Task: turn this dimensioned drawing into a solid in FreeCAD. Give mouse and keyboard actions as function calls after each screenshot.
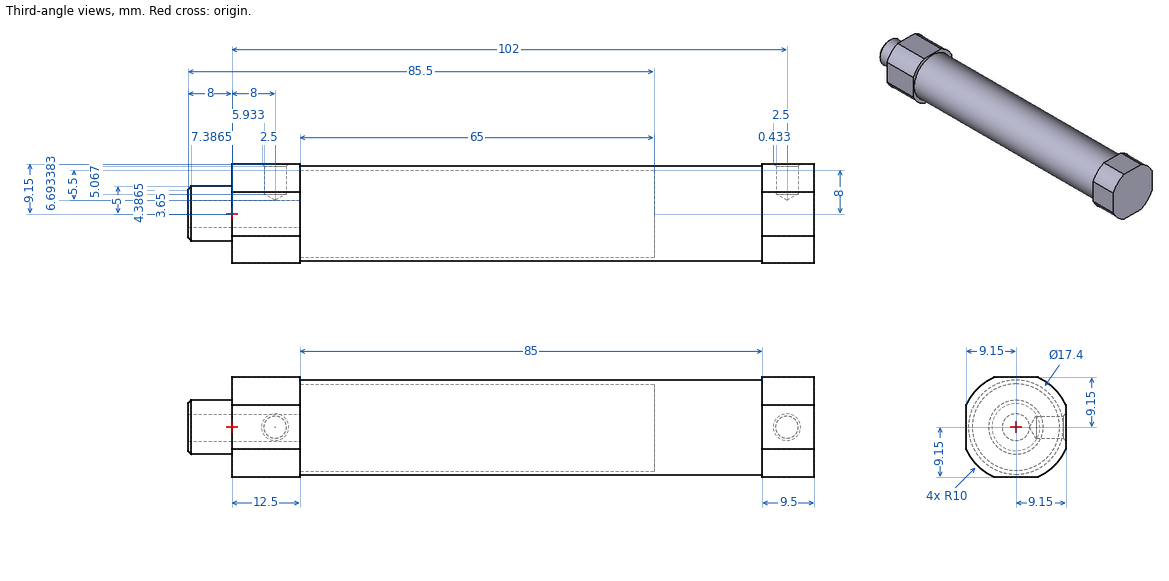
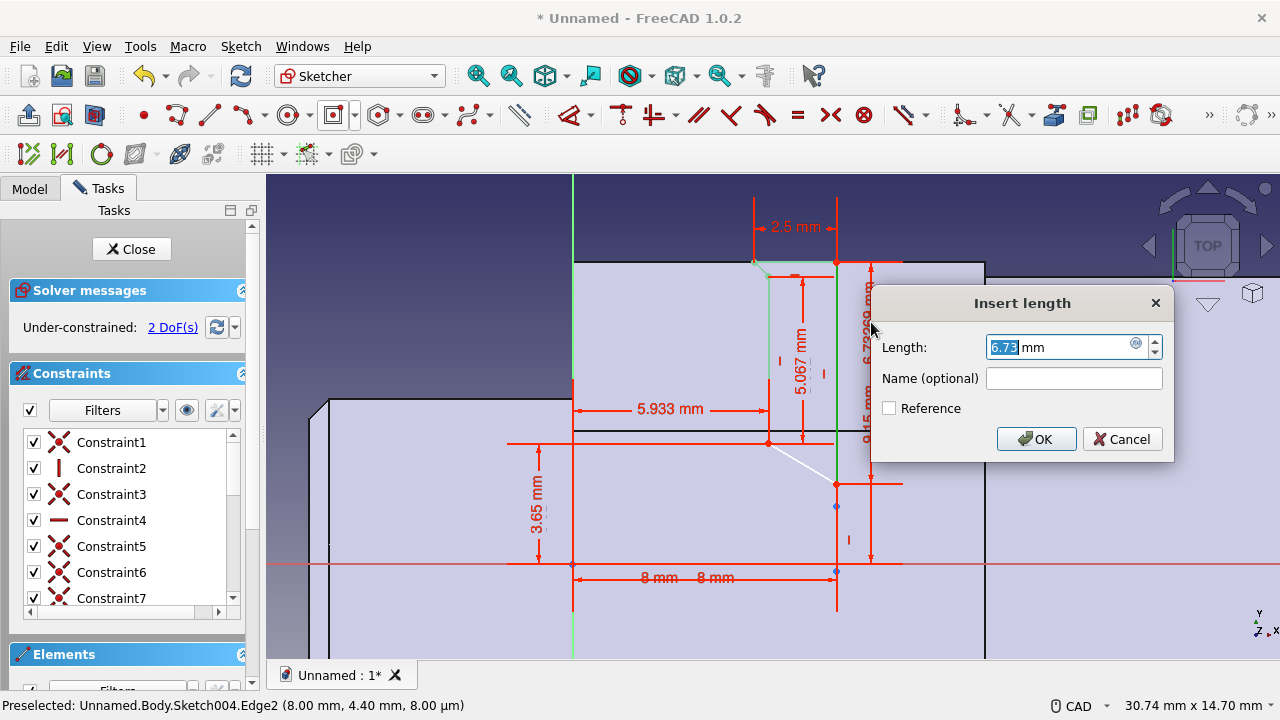
text(6.693383)
key(Return)
key(Escape)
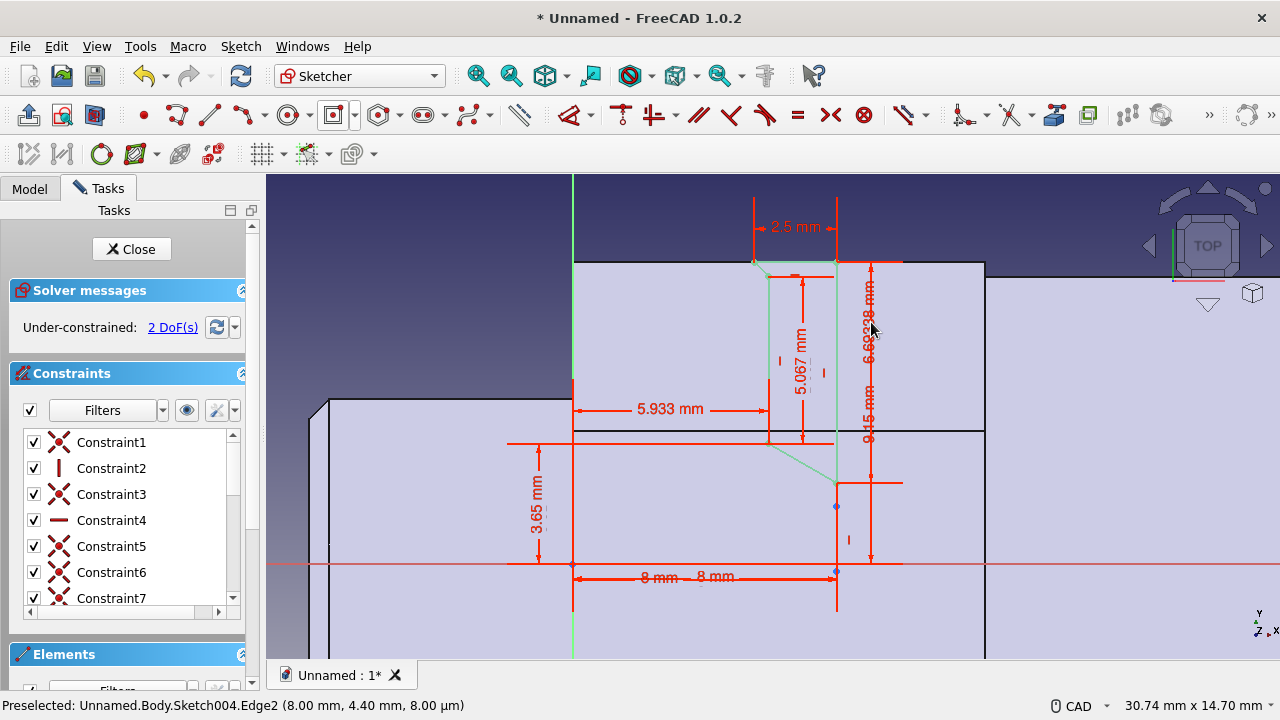
click(132, 249)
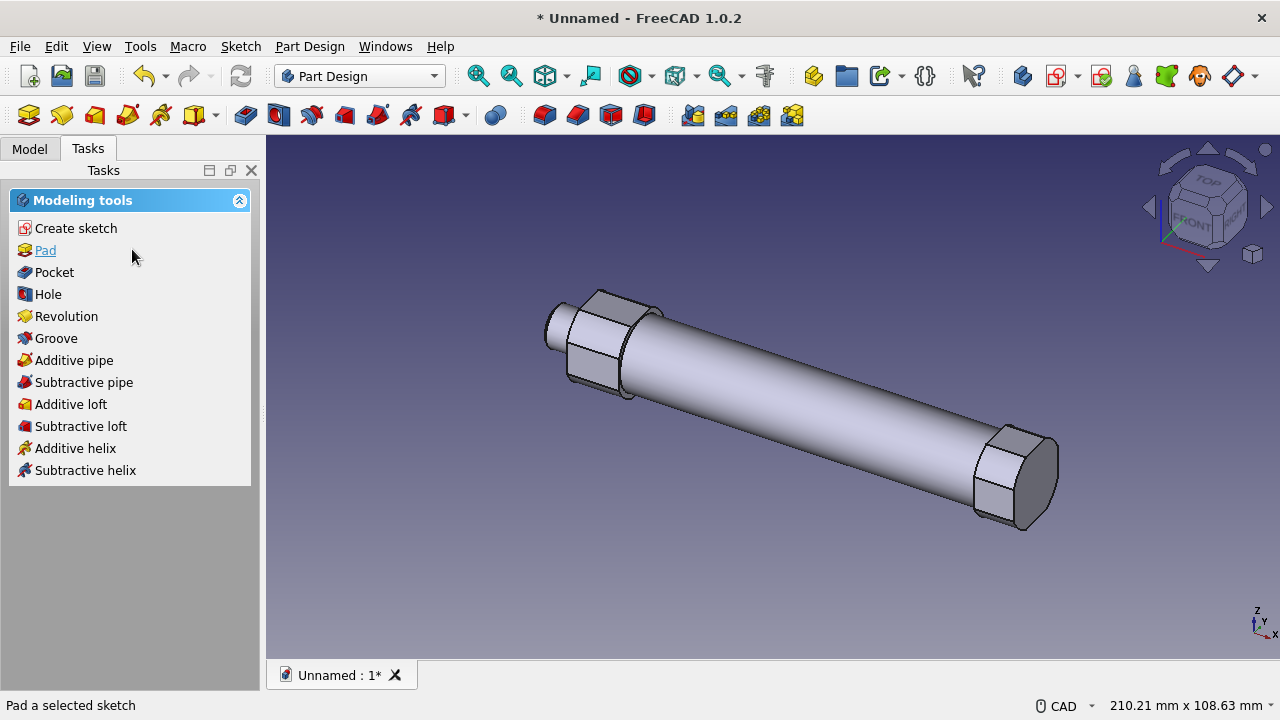
click(312, 116)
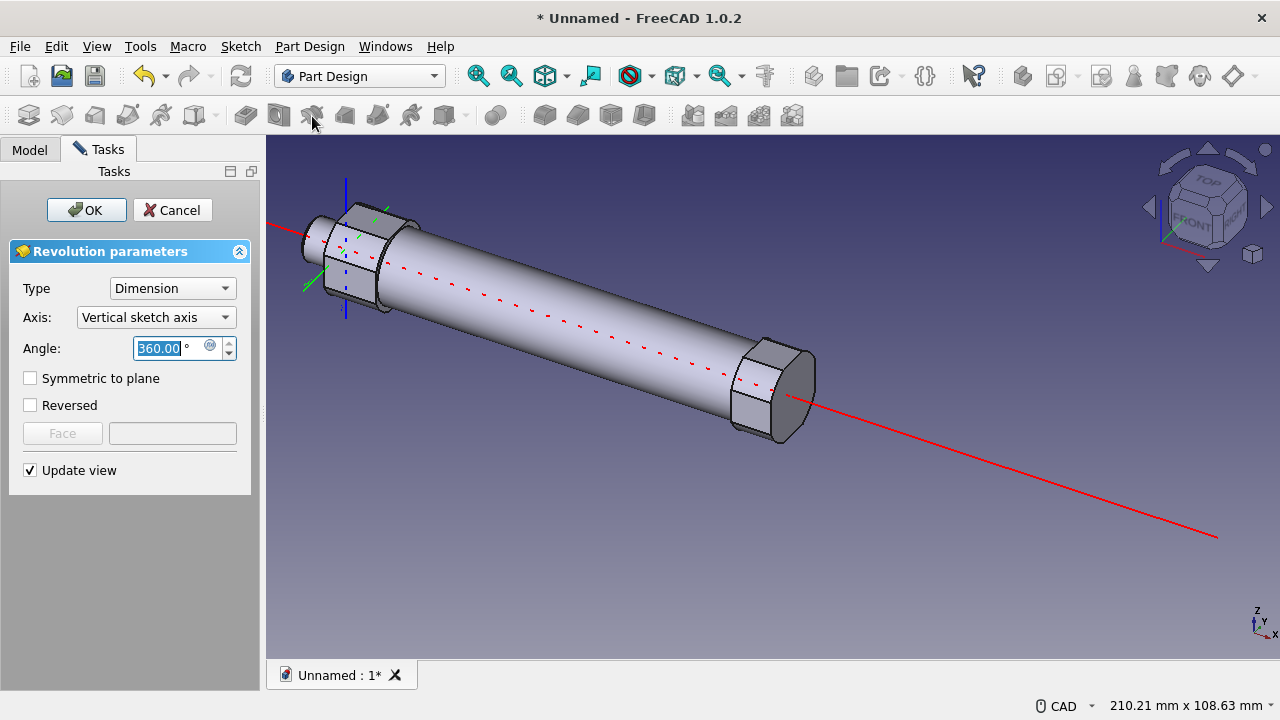
click(157, 318)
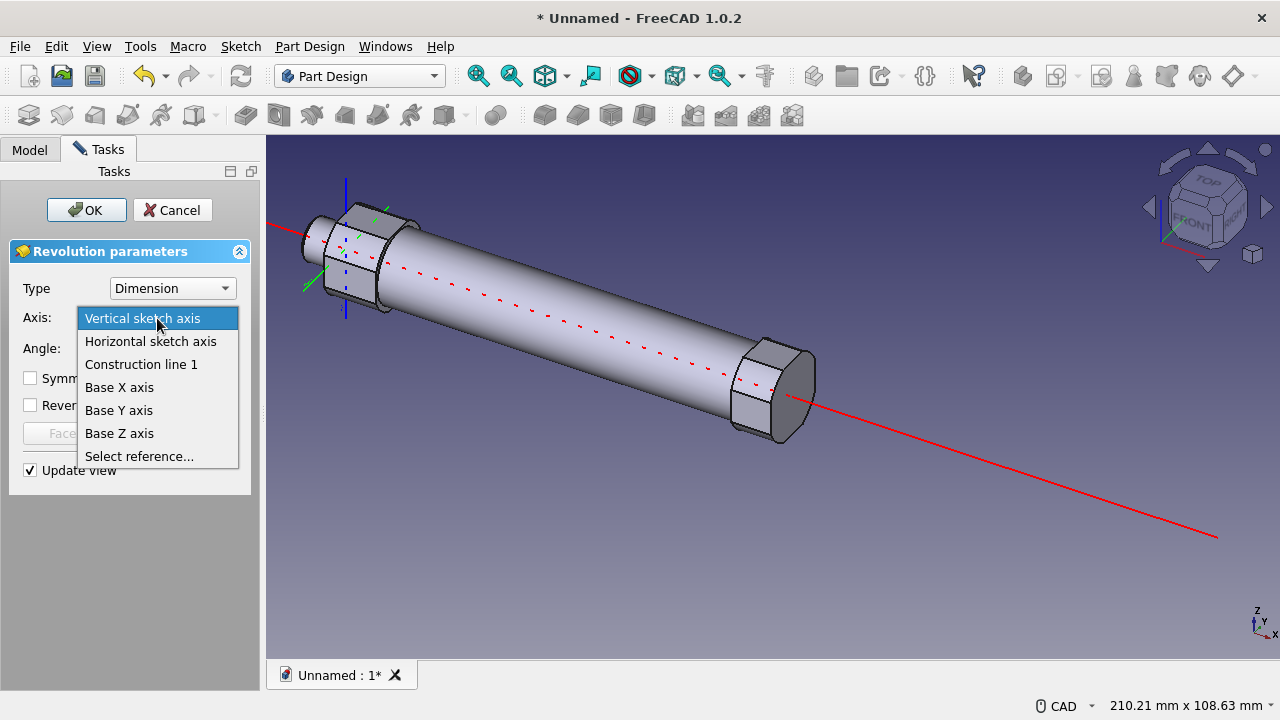
click(156, 364)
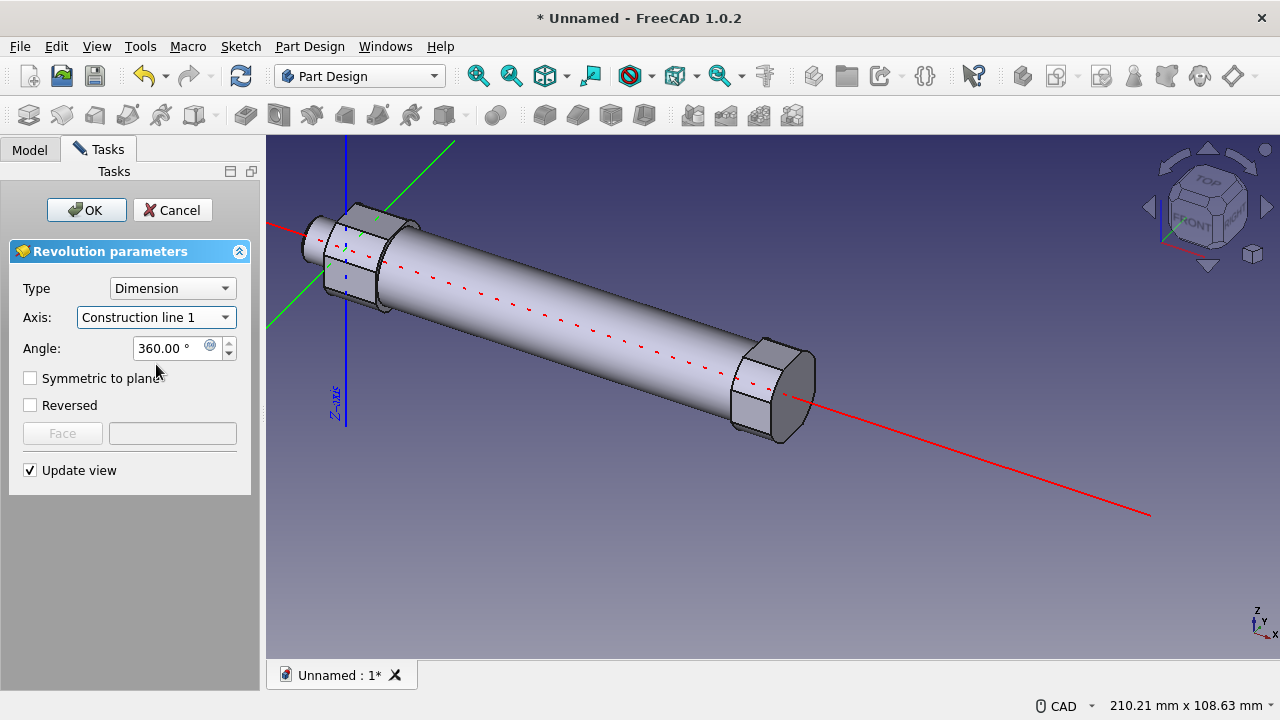
click(87, 210)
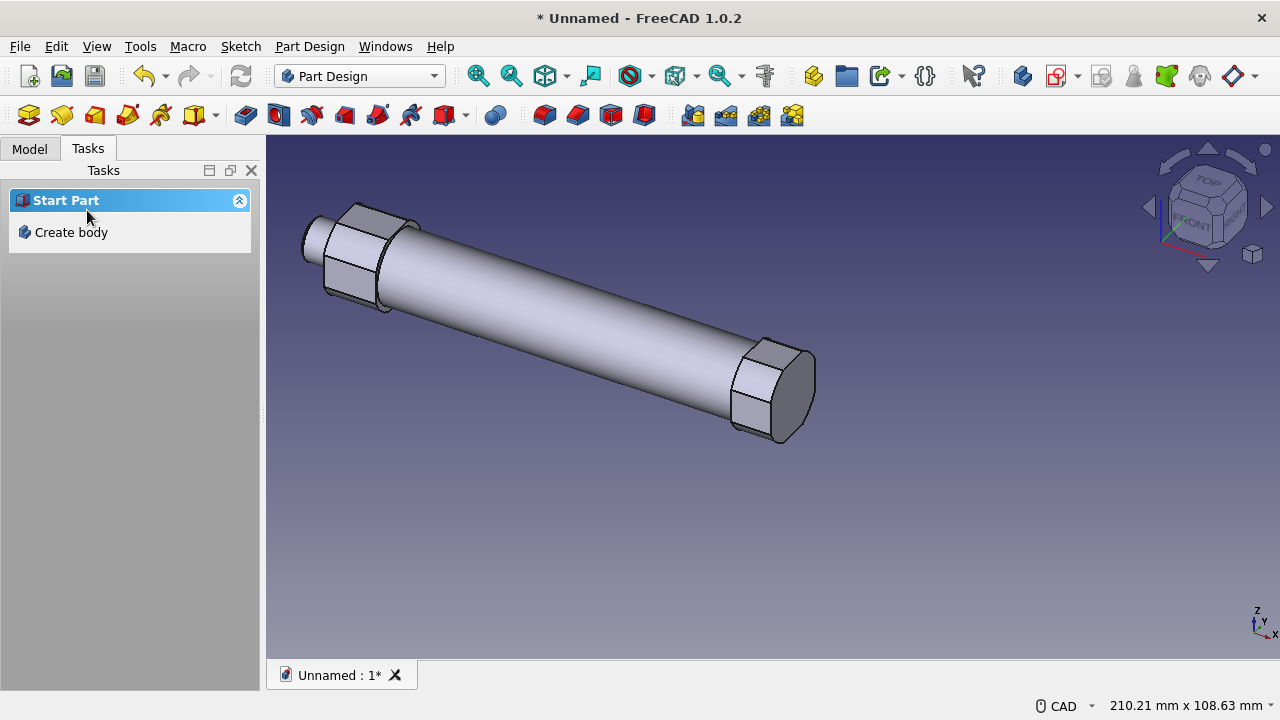
click(1056, 76)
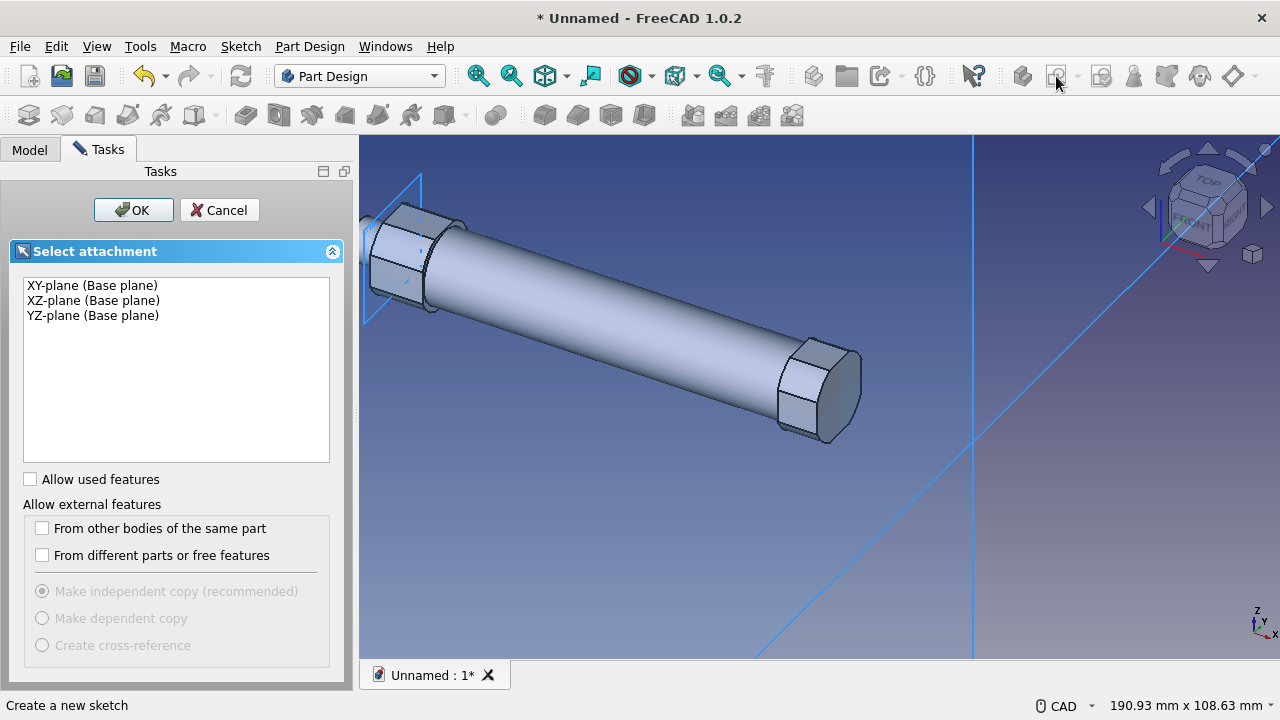
click(84, 286)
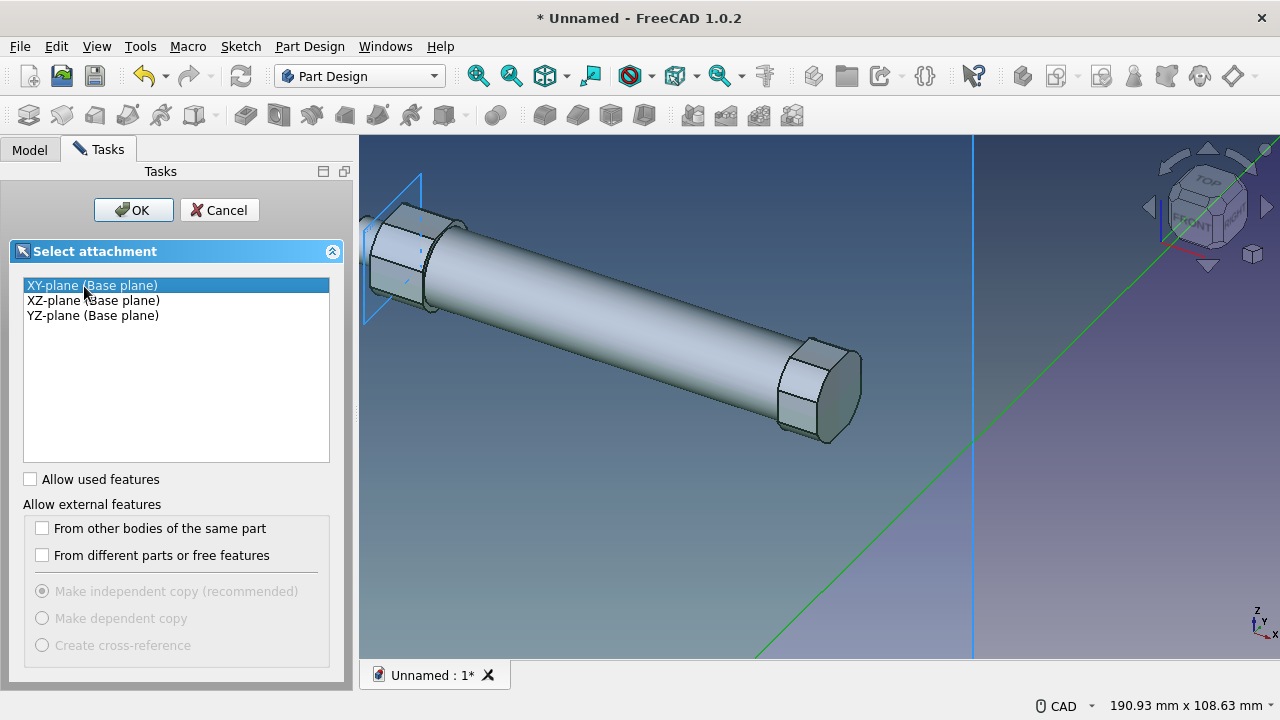
click(134, 210)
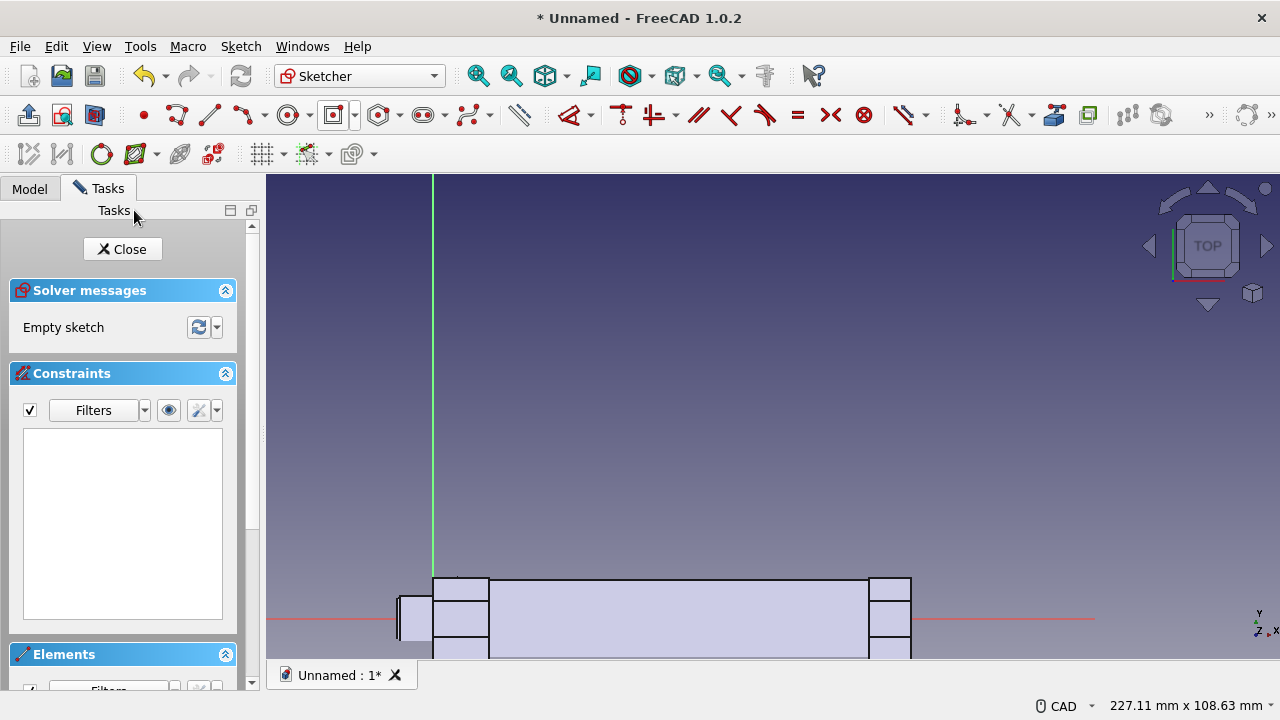
click(95, 116)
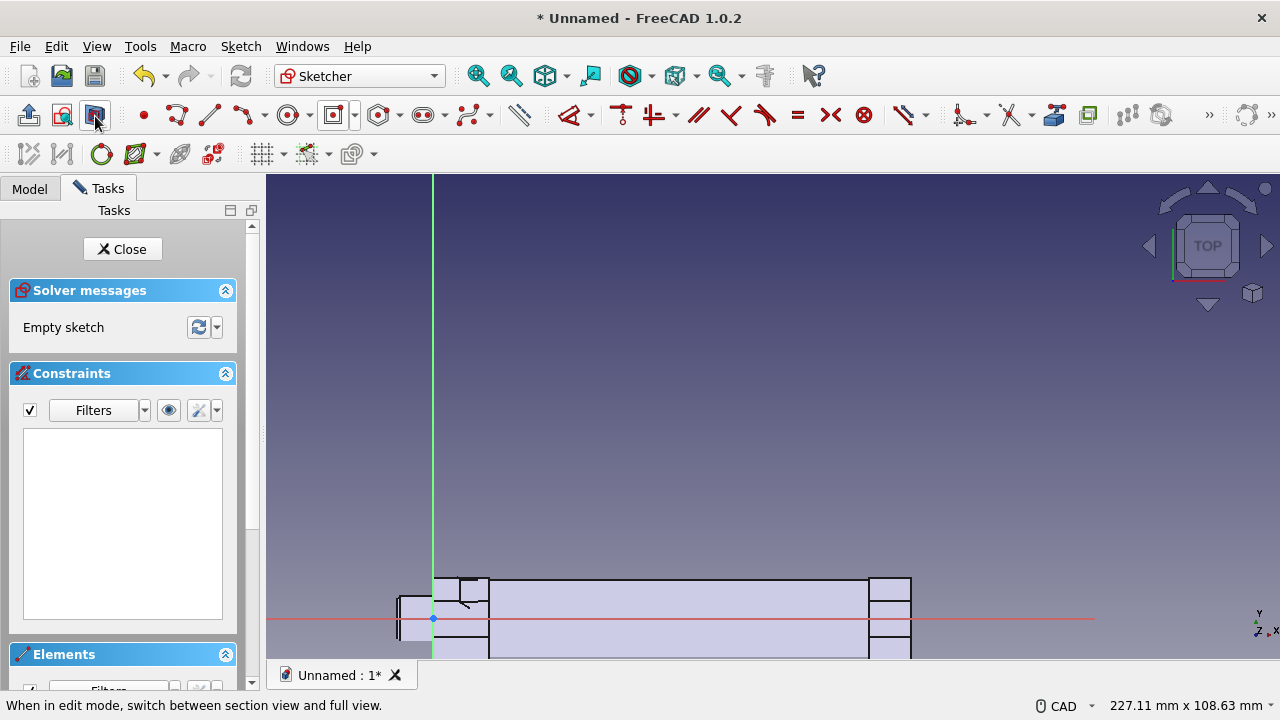
scroll(911, 627, up, 10)